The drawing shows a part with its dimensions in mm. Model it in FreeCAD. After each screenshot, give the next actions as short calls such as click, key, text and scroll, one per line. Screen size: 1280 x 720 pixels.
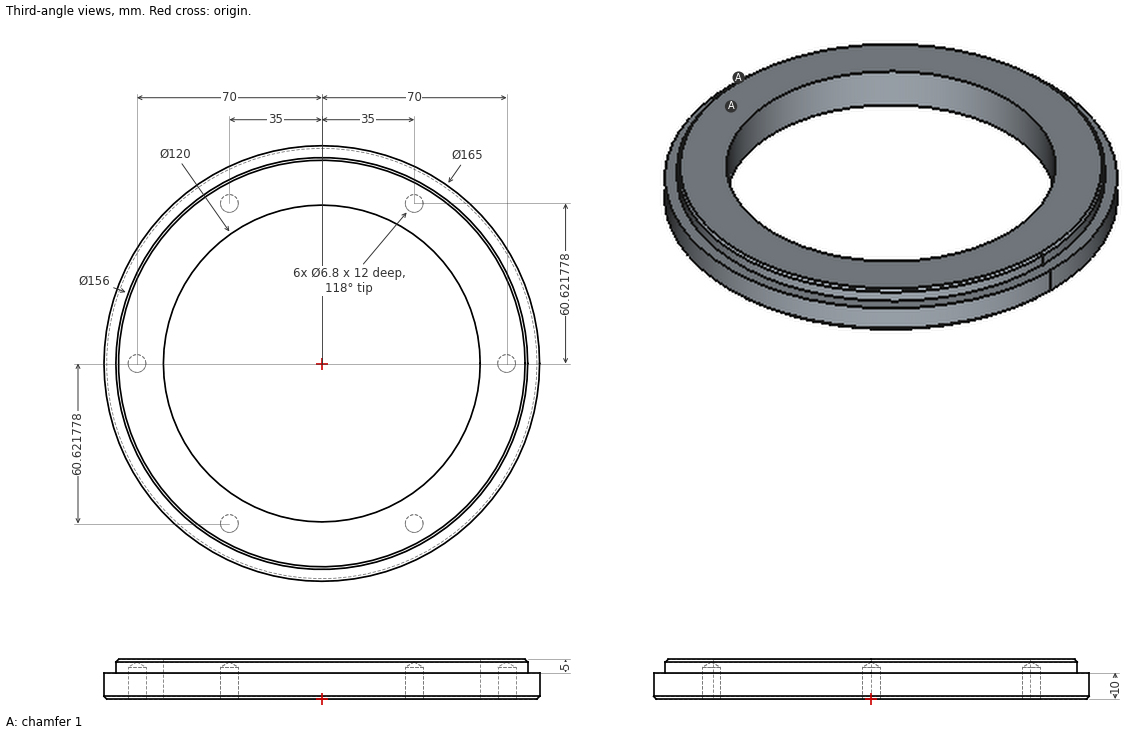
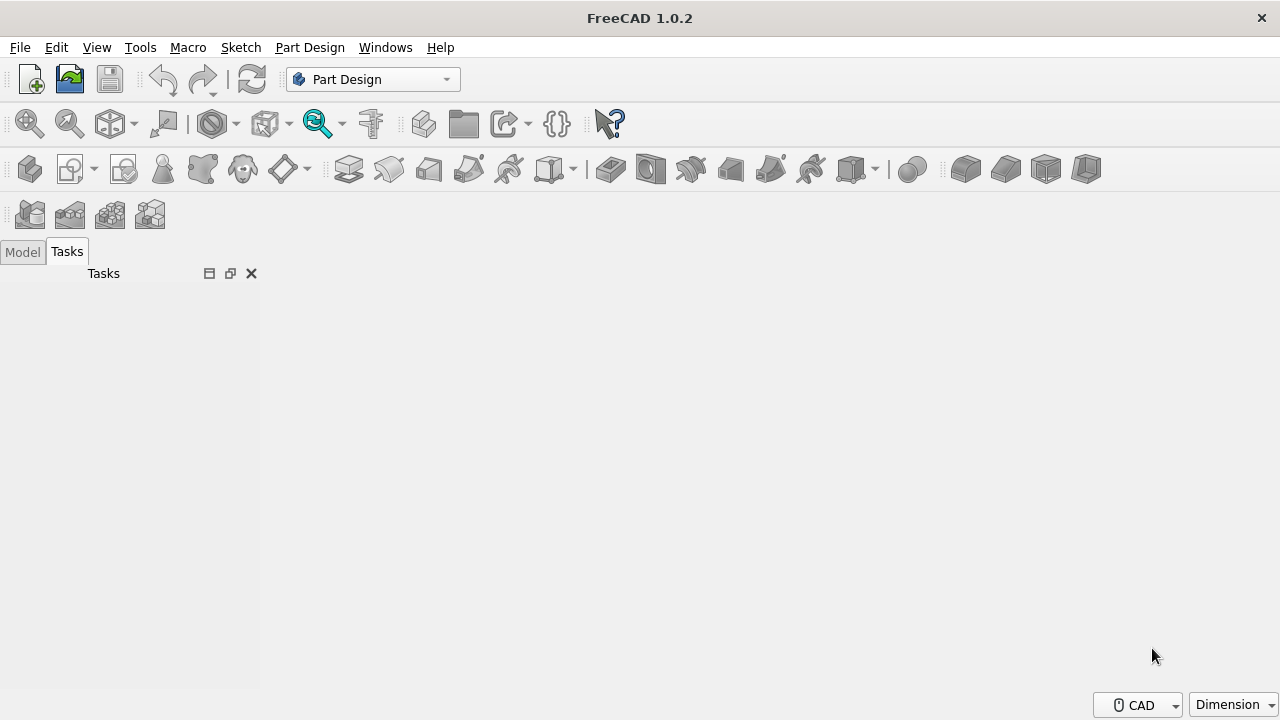
click(30, 80)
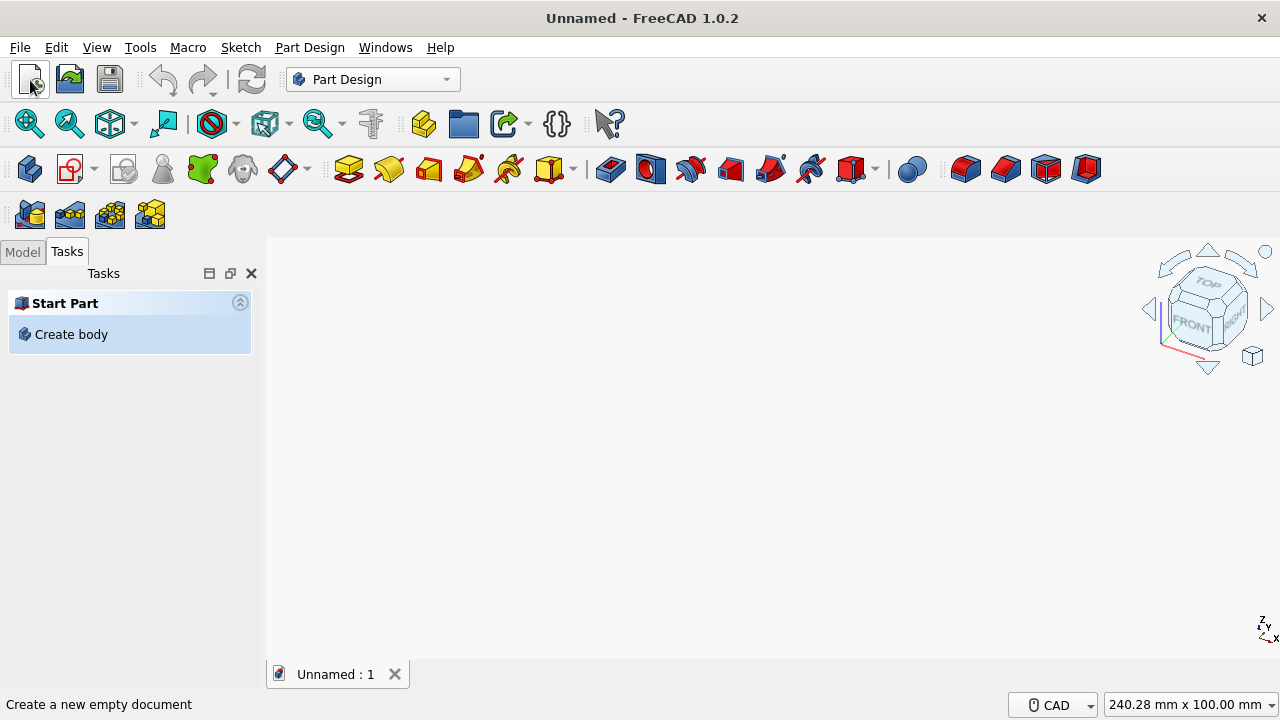
click(70, 170)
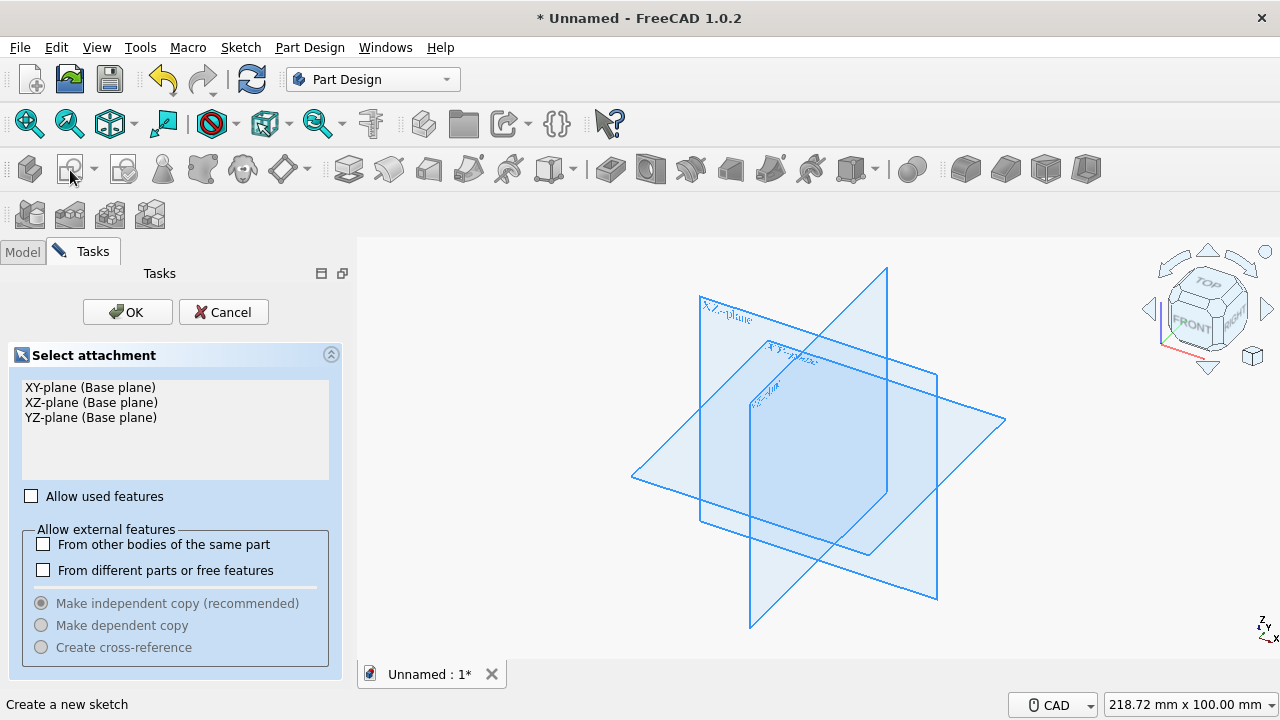
click(82, 388)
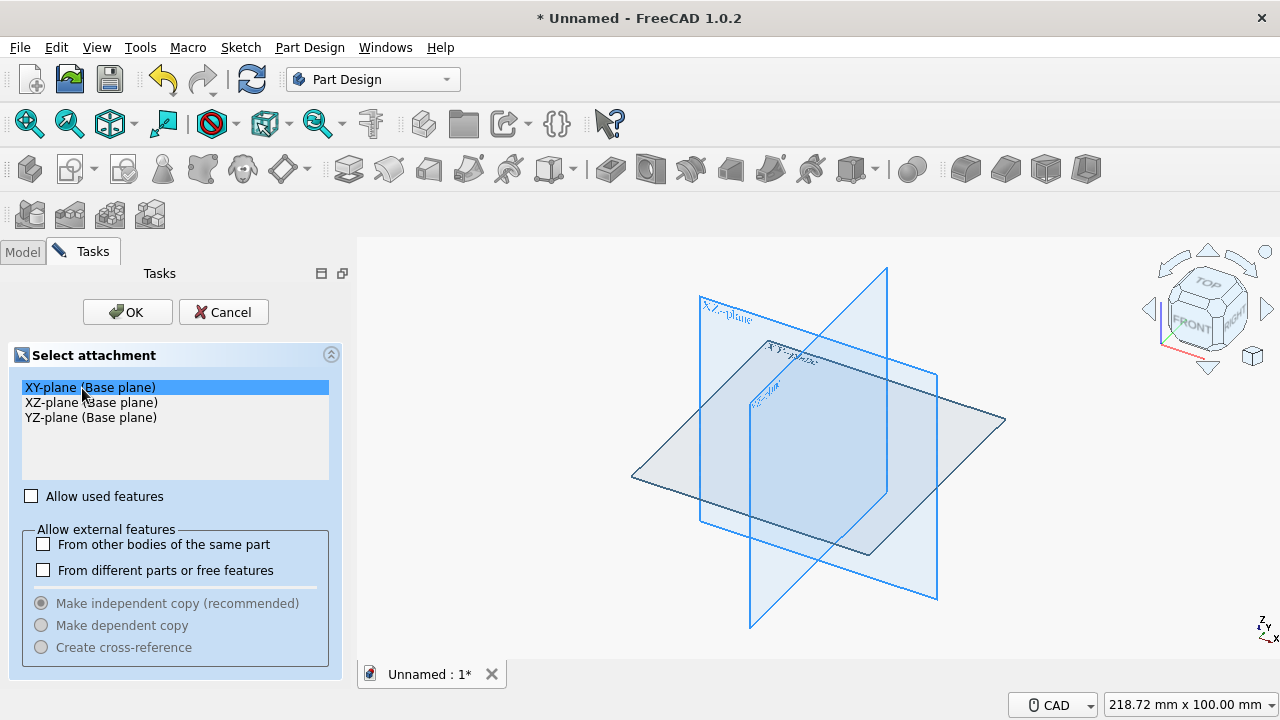
click(128, 312)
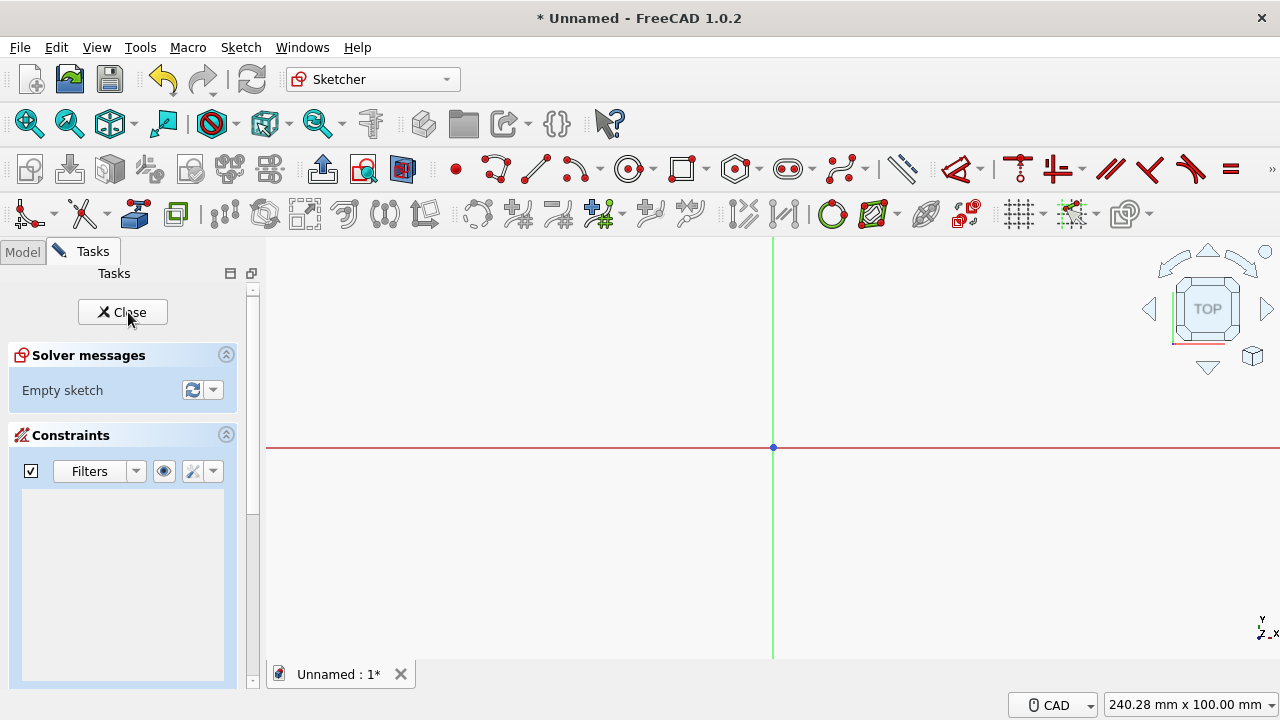
scroll(665, 448, down, 5)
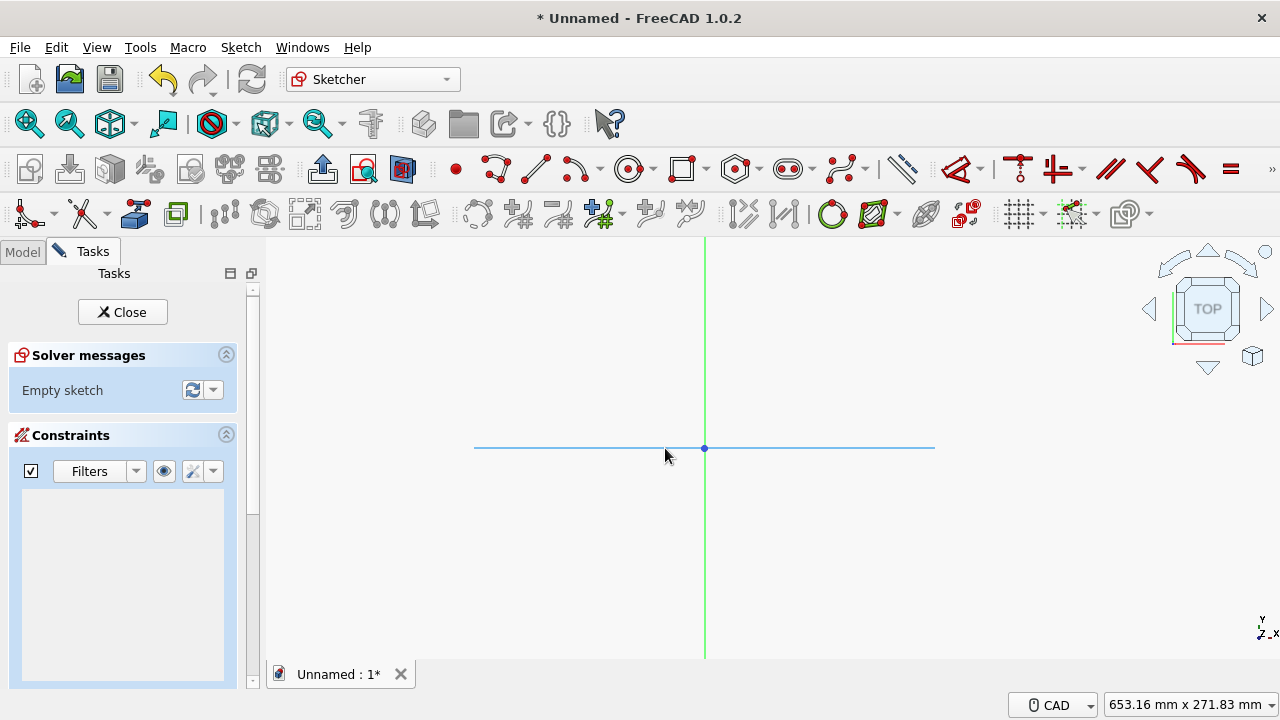
click(630, 170)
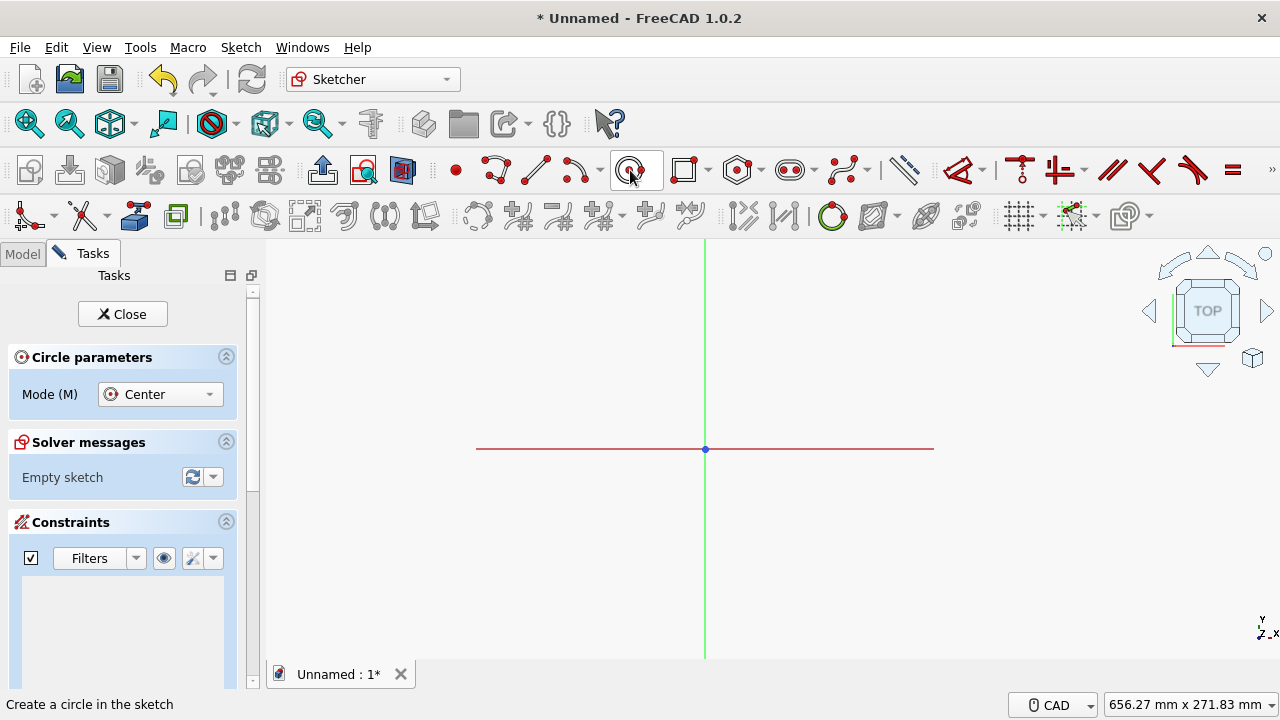
click(705, 449)
move(795, 359)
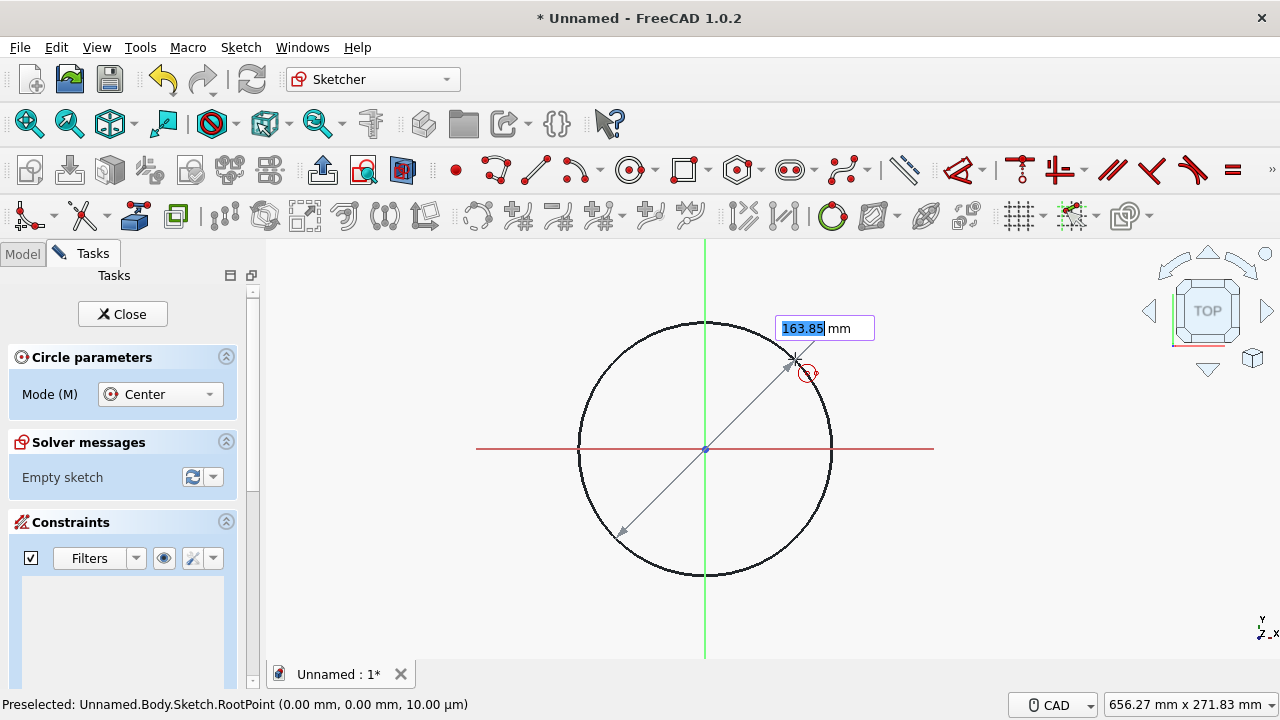
text(165)
key(Return)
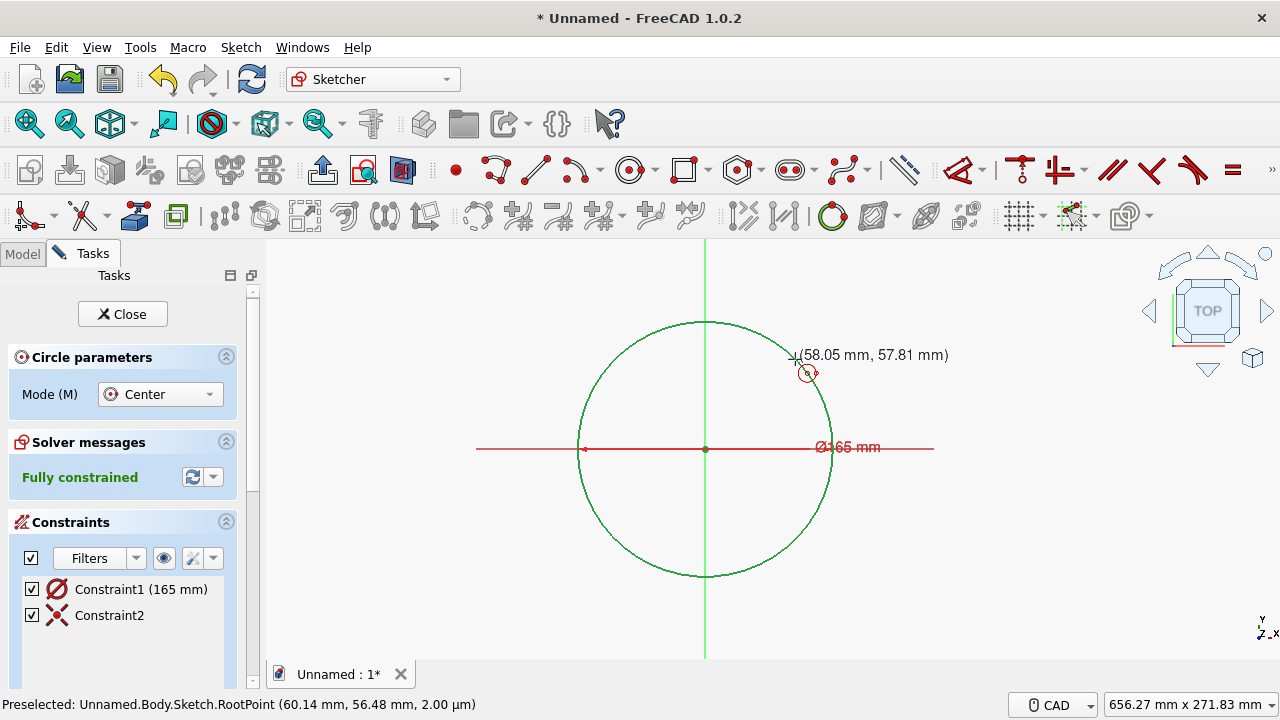
click(705, 449)
move(771, 384)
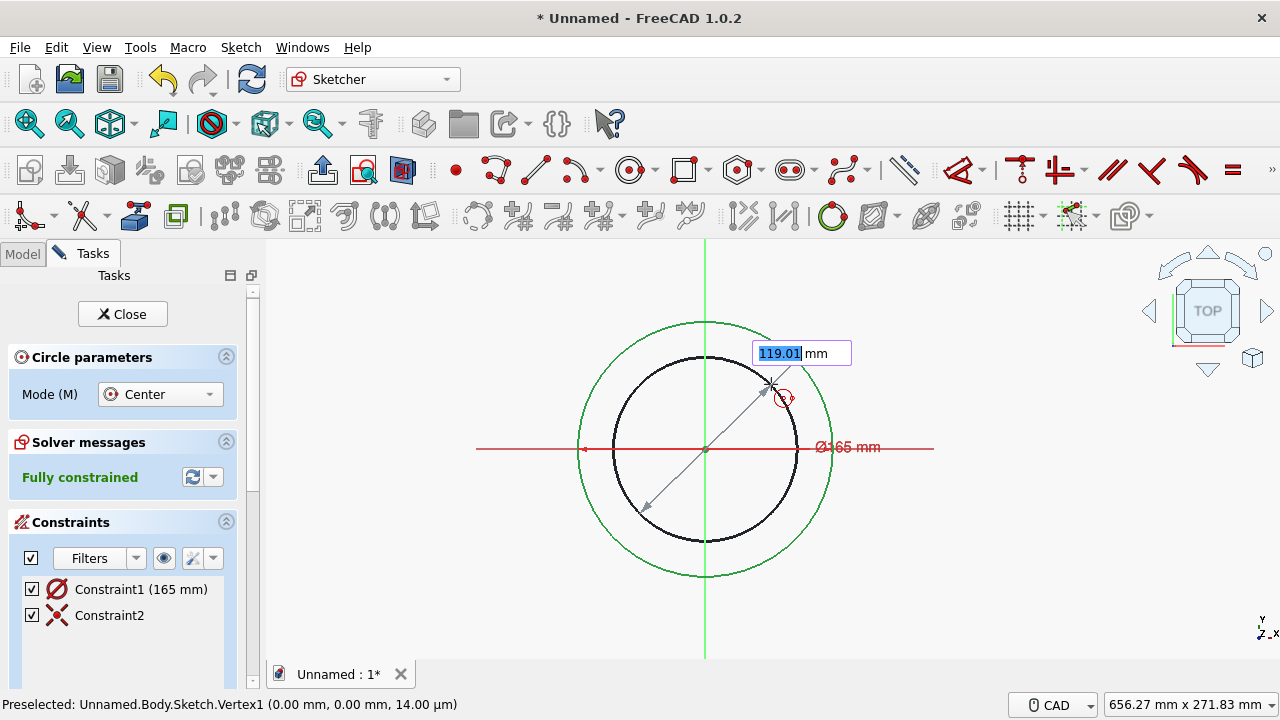
text(120)
key(Return)
key(Escape)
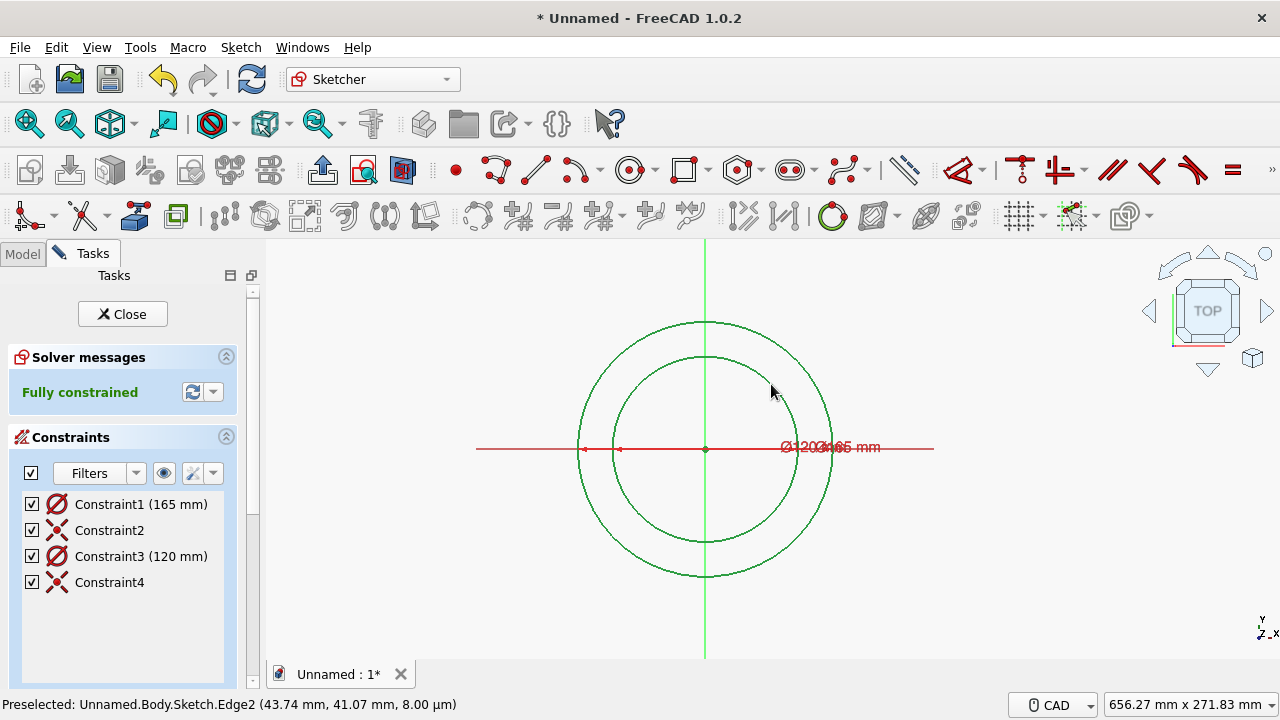
click(123, 314)